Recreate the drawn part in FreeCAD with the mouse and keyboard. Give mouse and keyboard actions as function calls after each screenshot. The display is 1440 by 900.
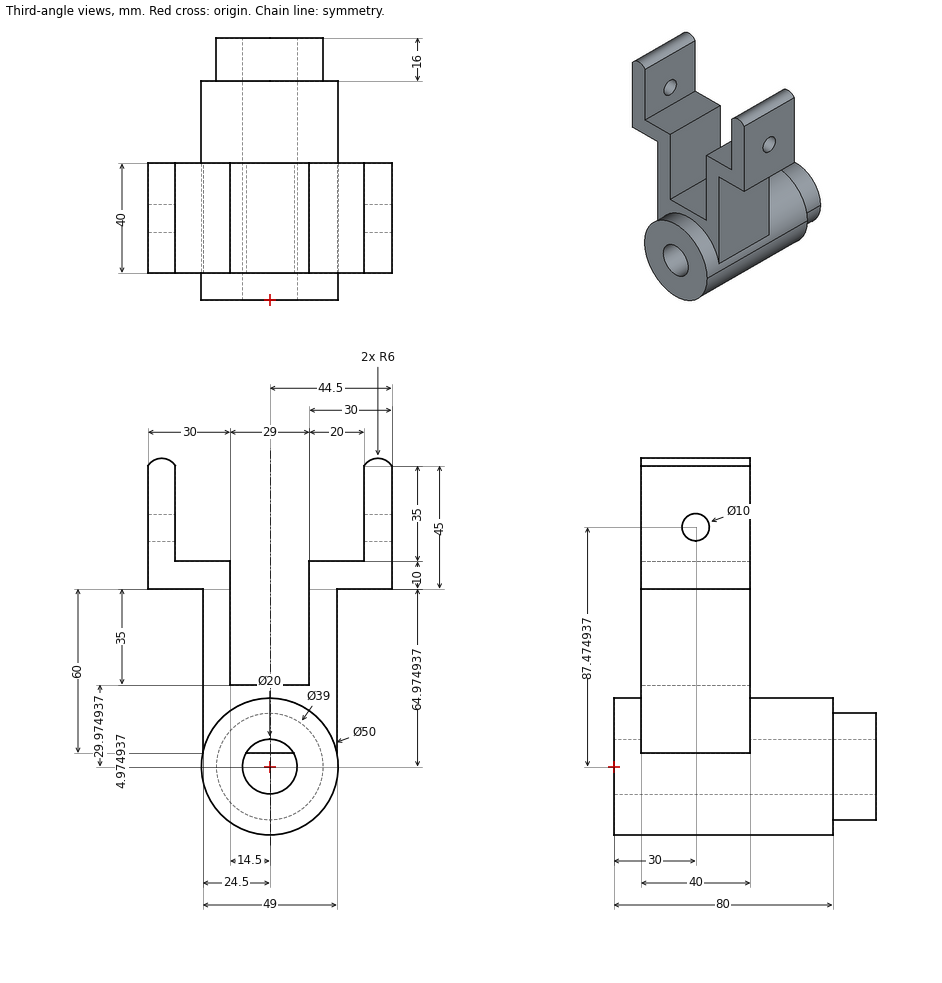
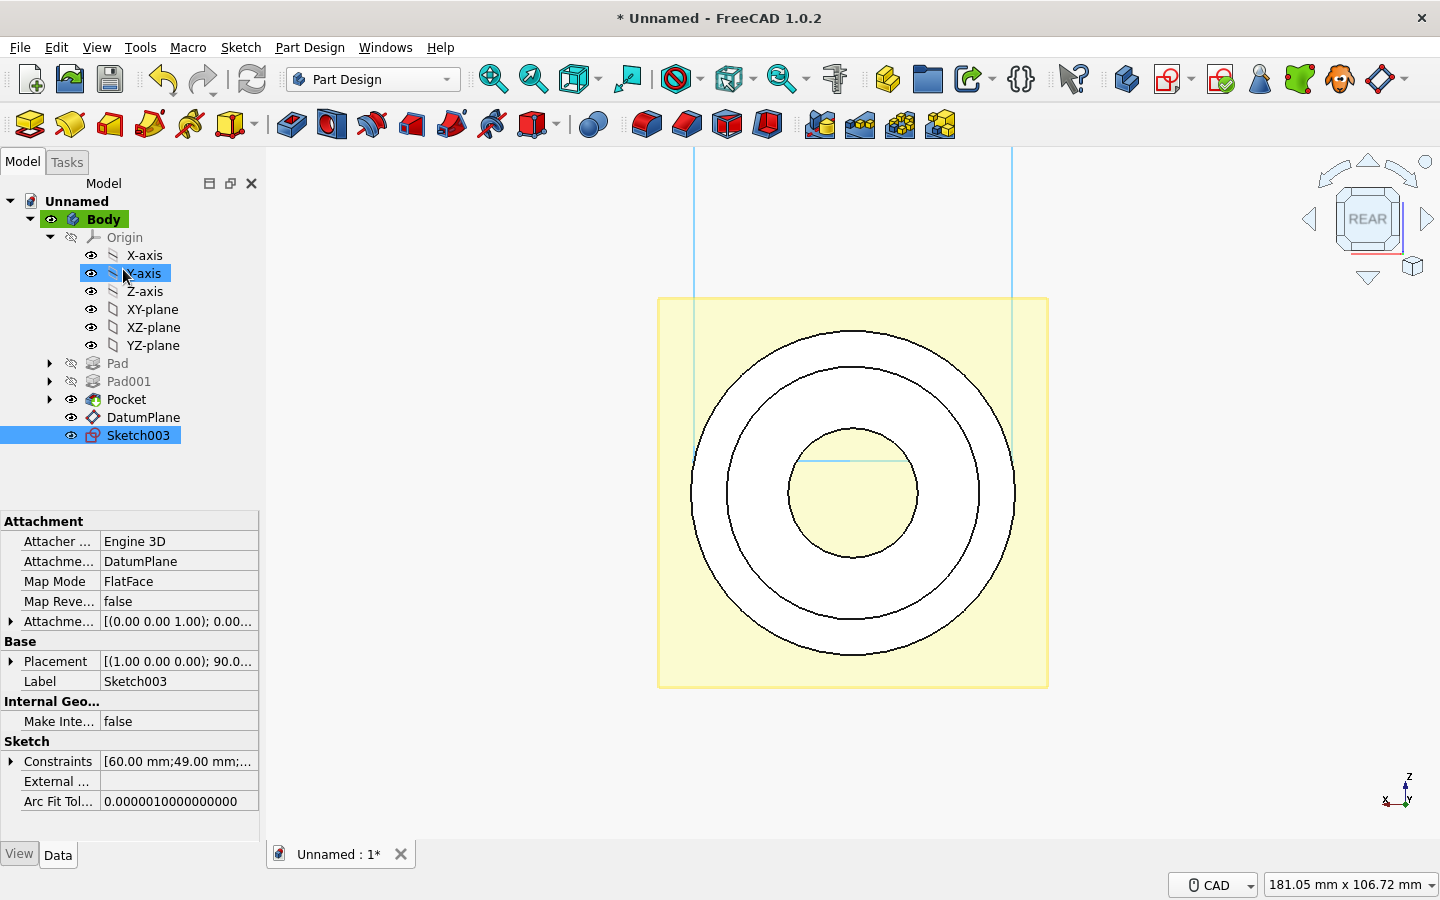
click(30, 124)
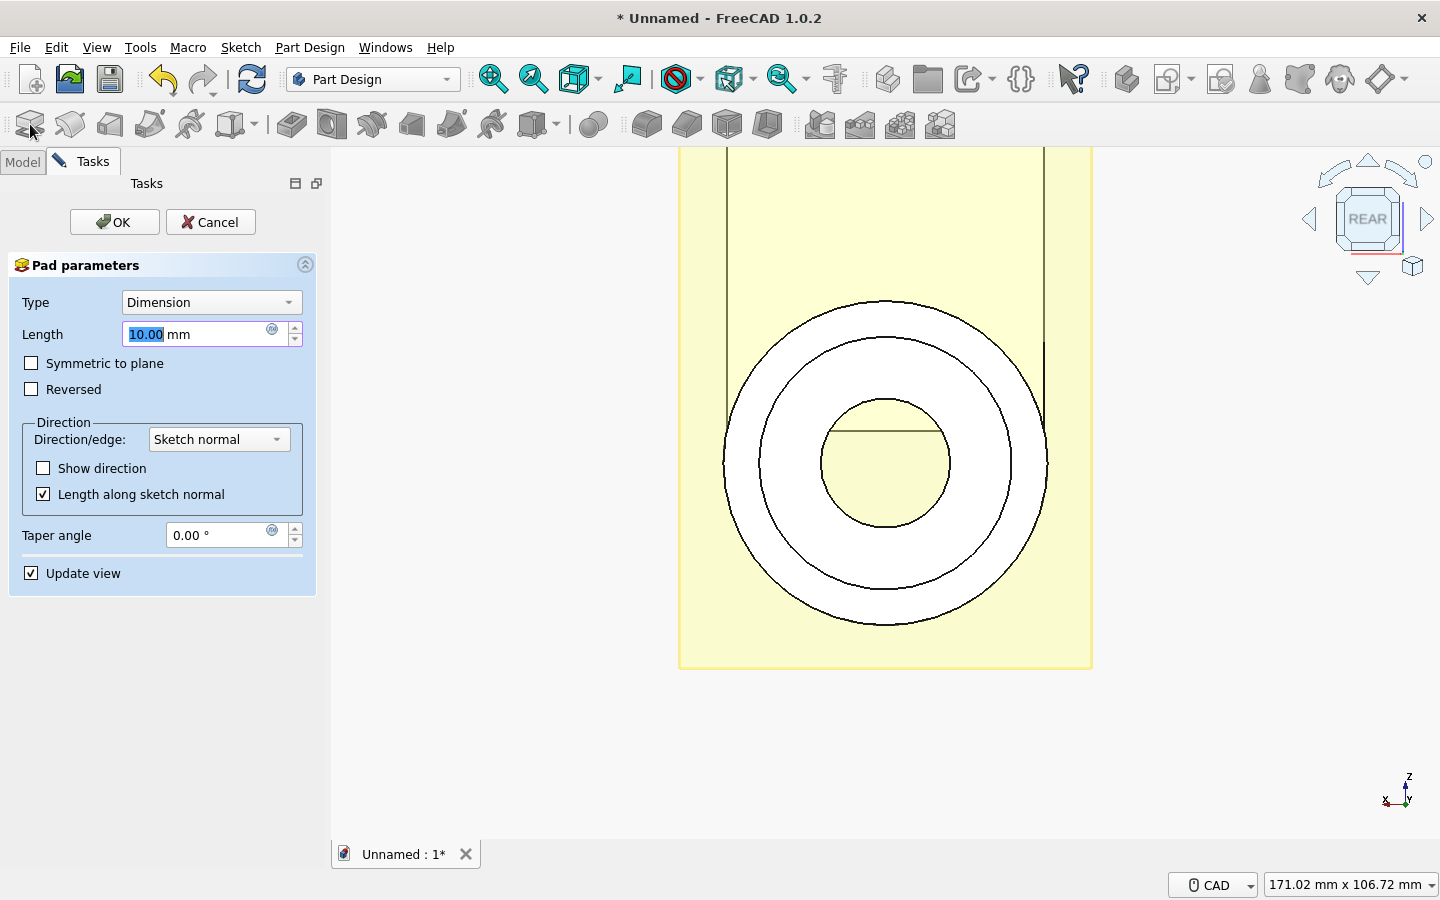
text(40)
key(Tab)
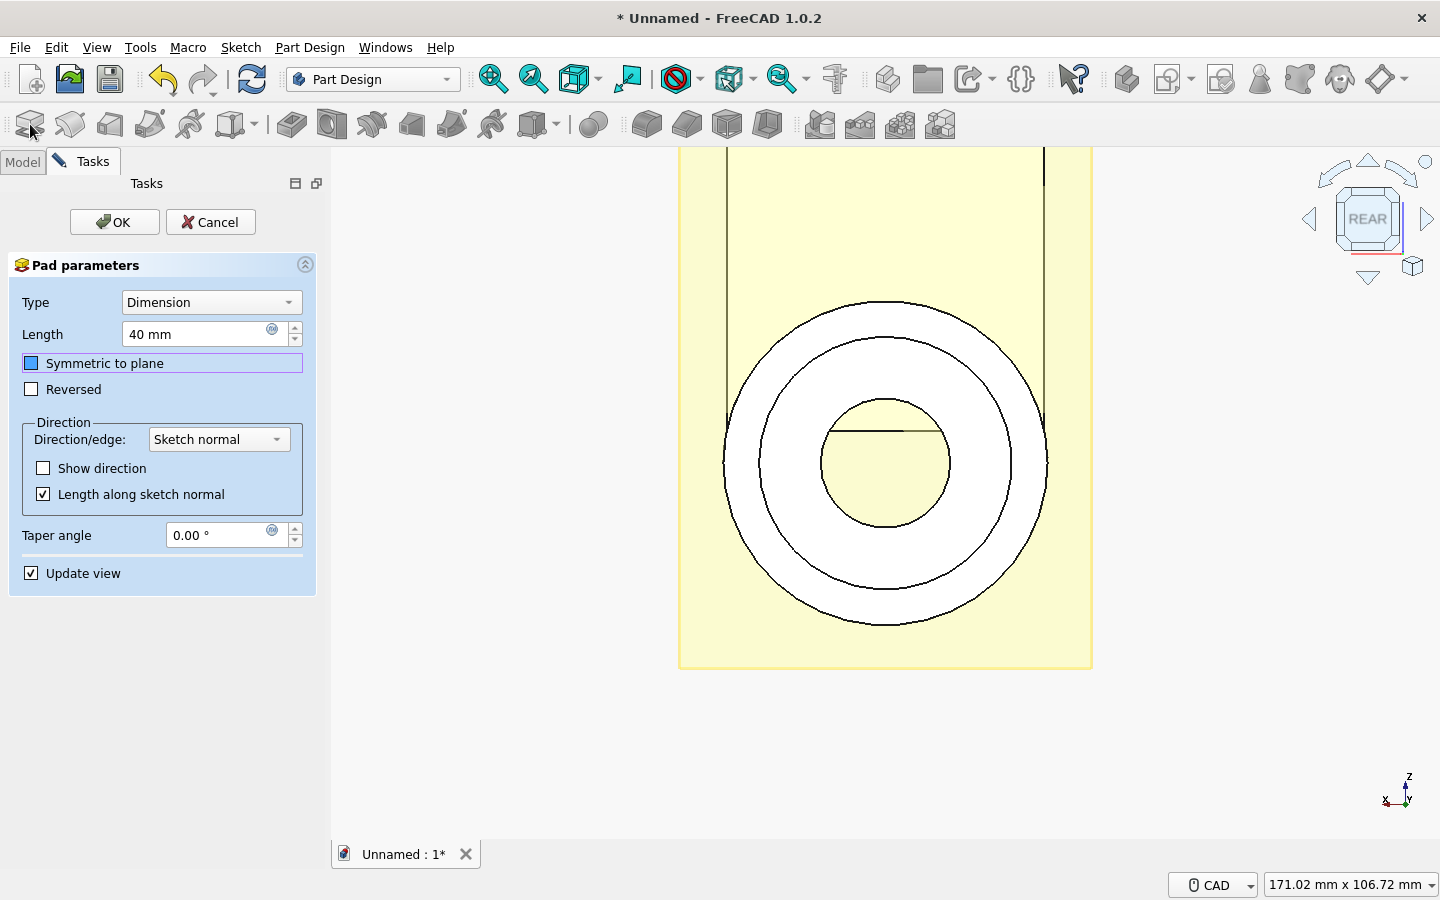
click(30, 389)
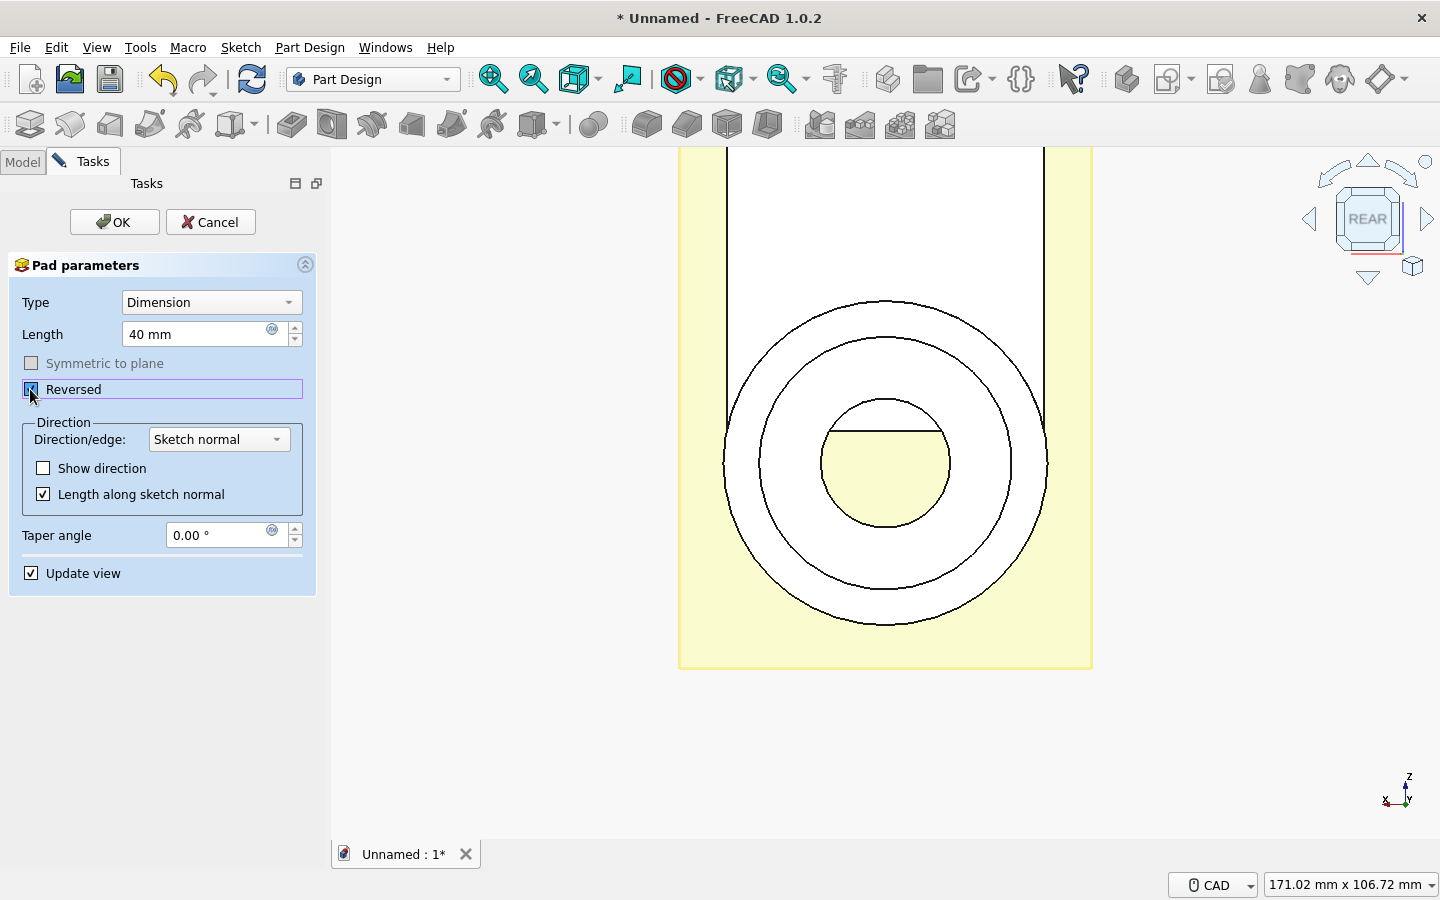
click(115, 222)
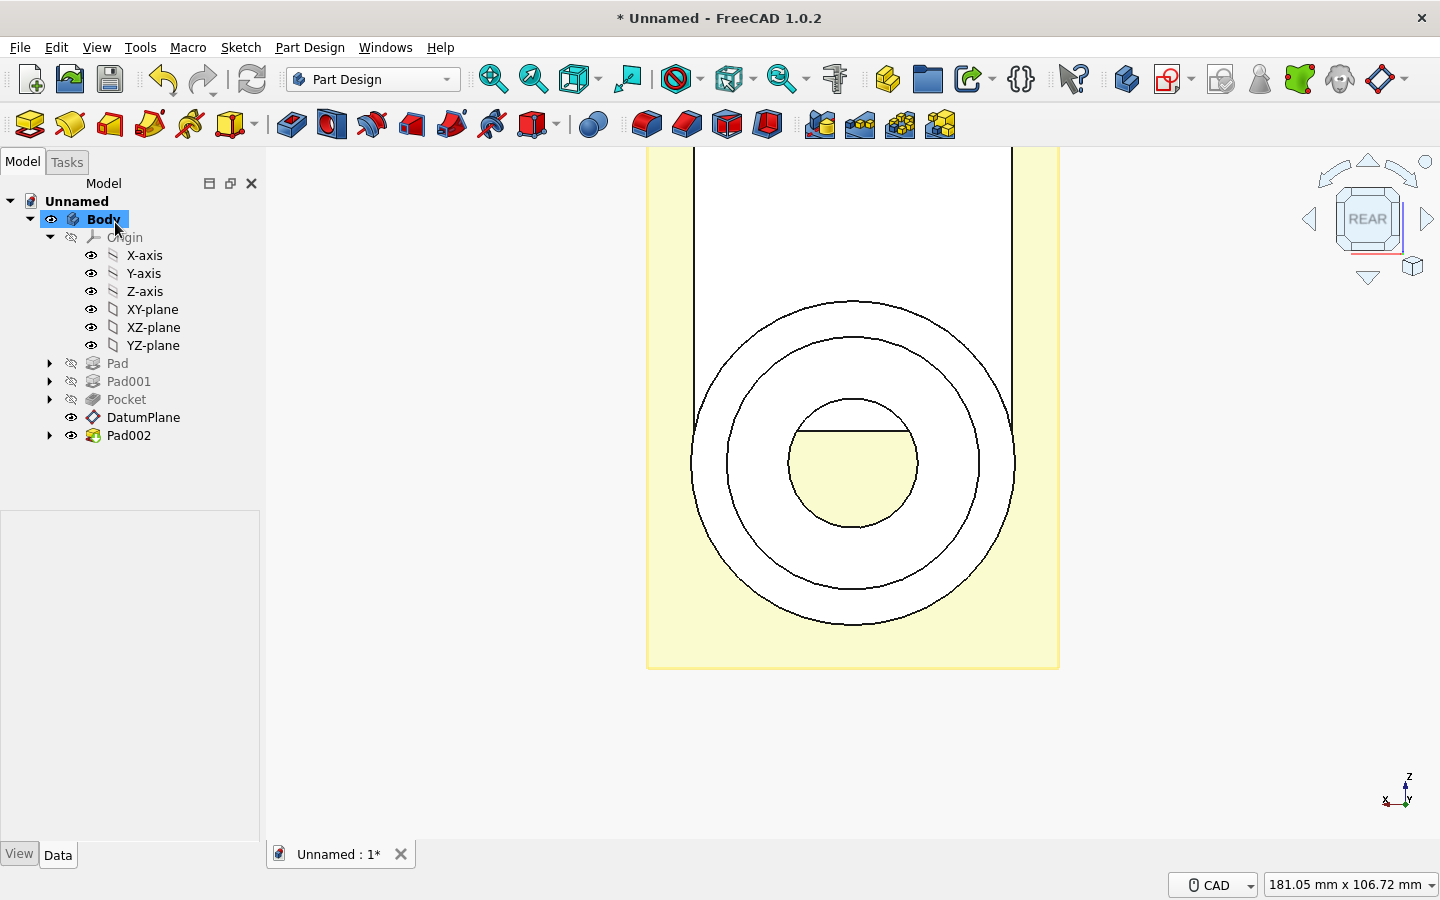
click(116, 417)
key(space)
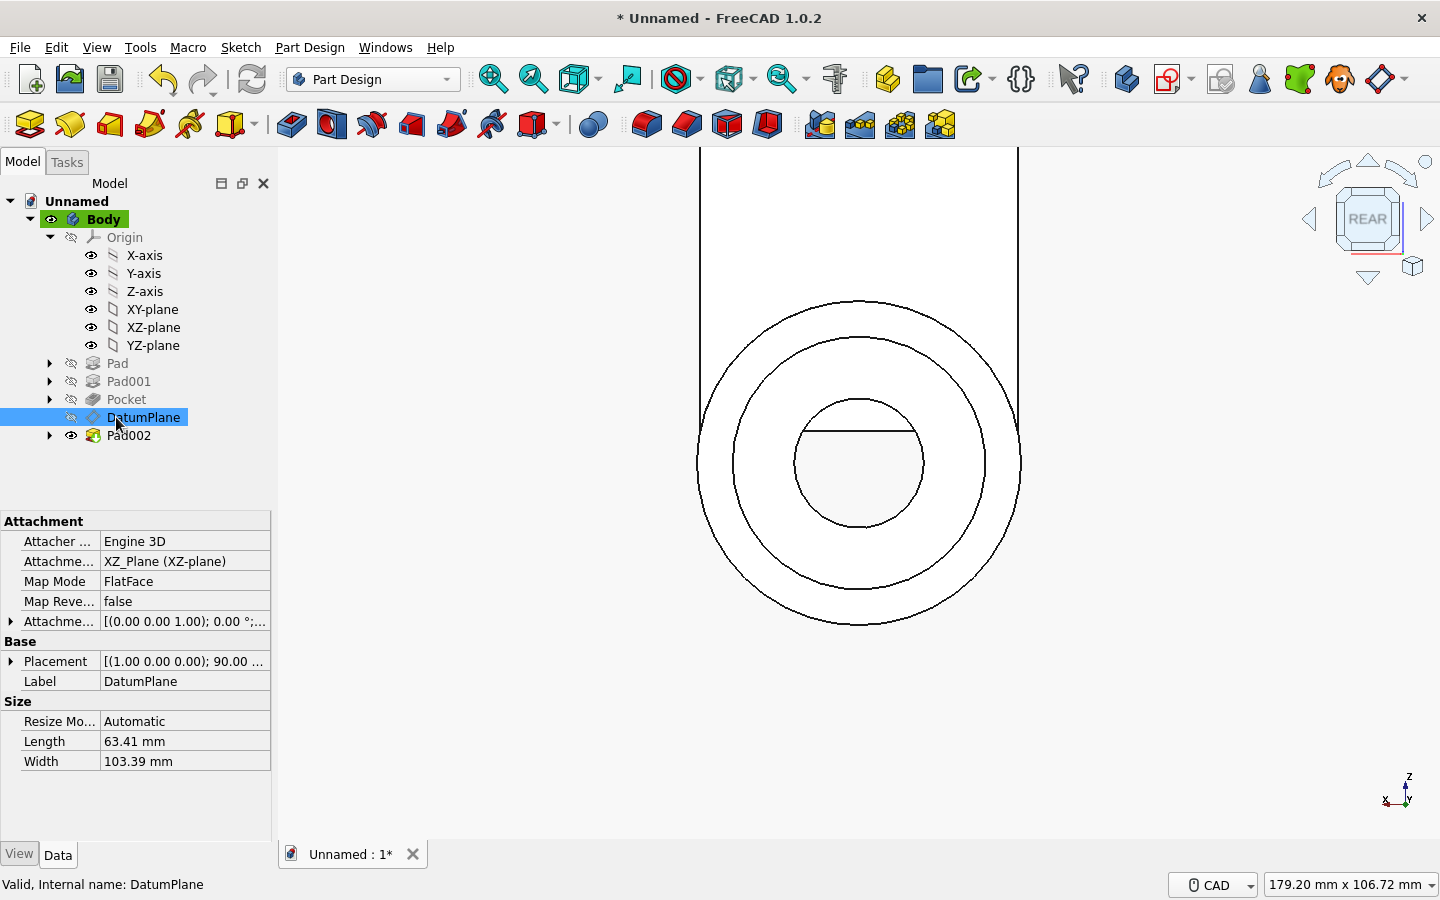
click(494, 80)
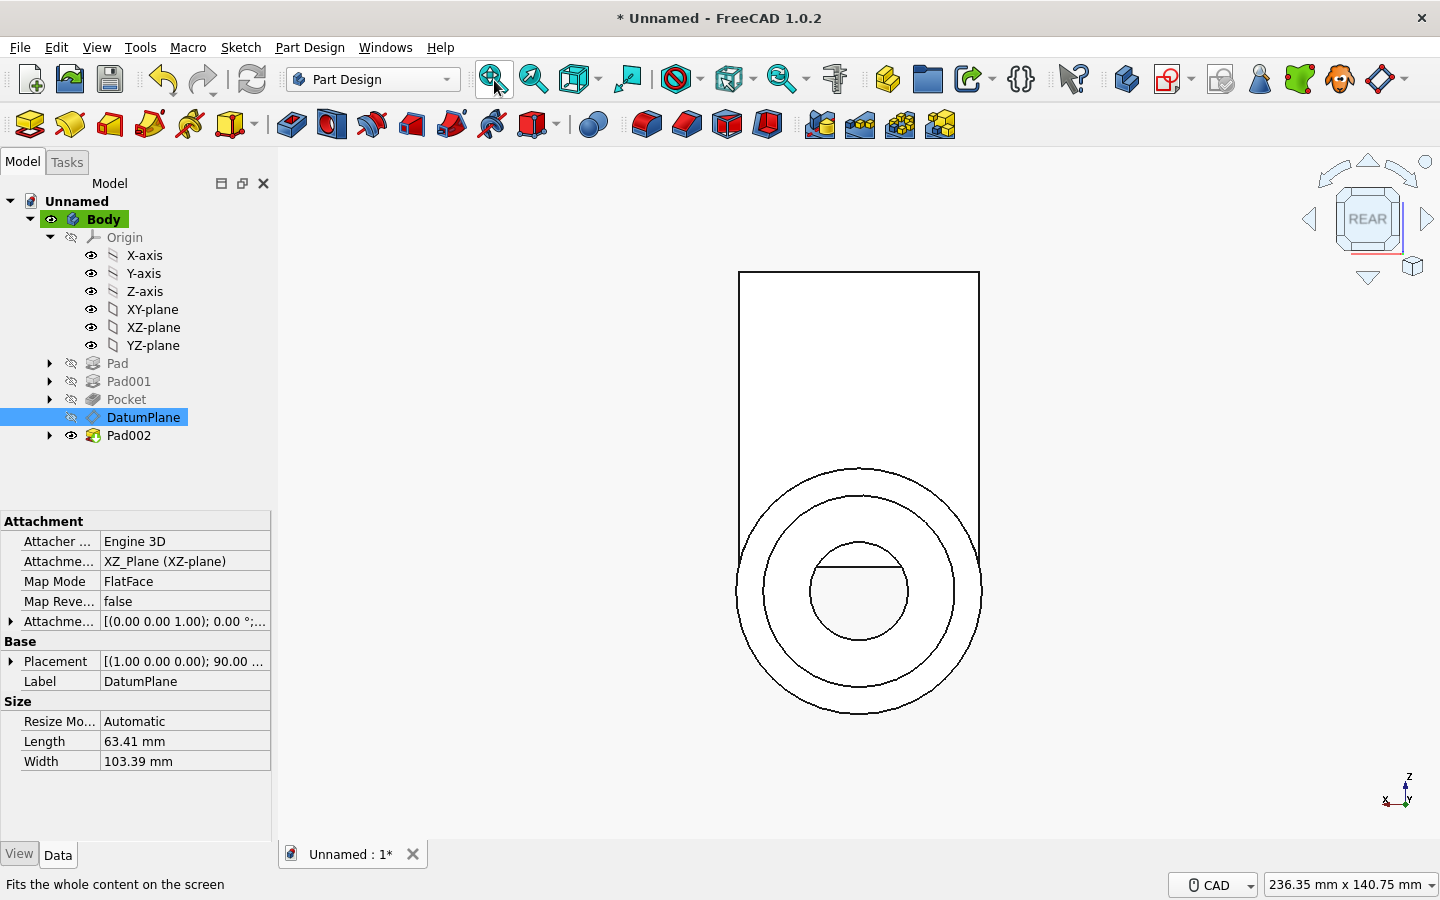
click(859, 376)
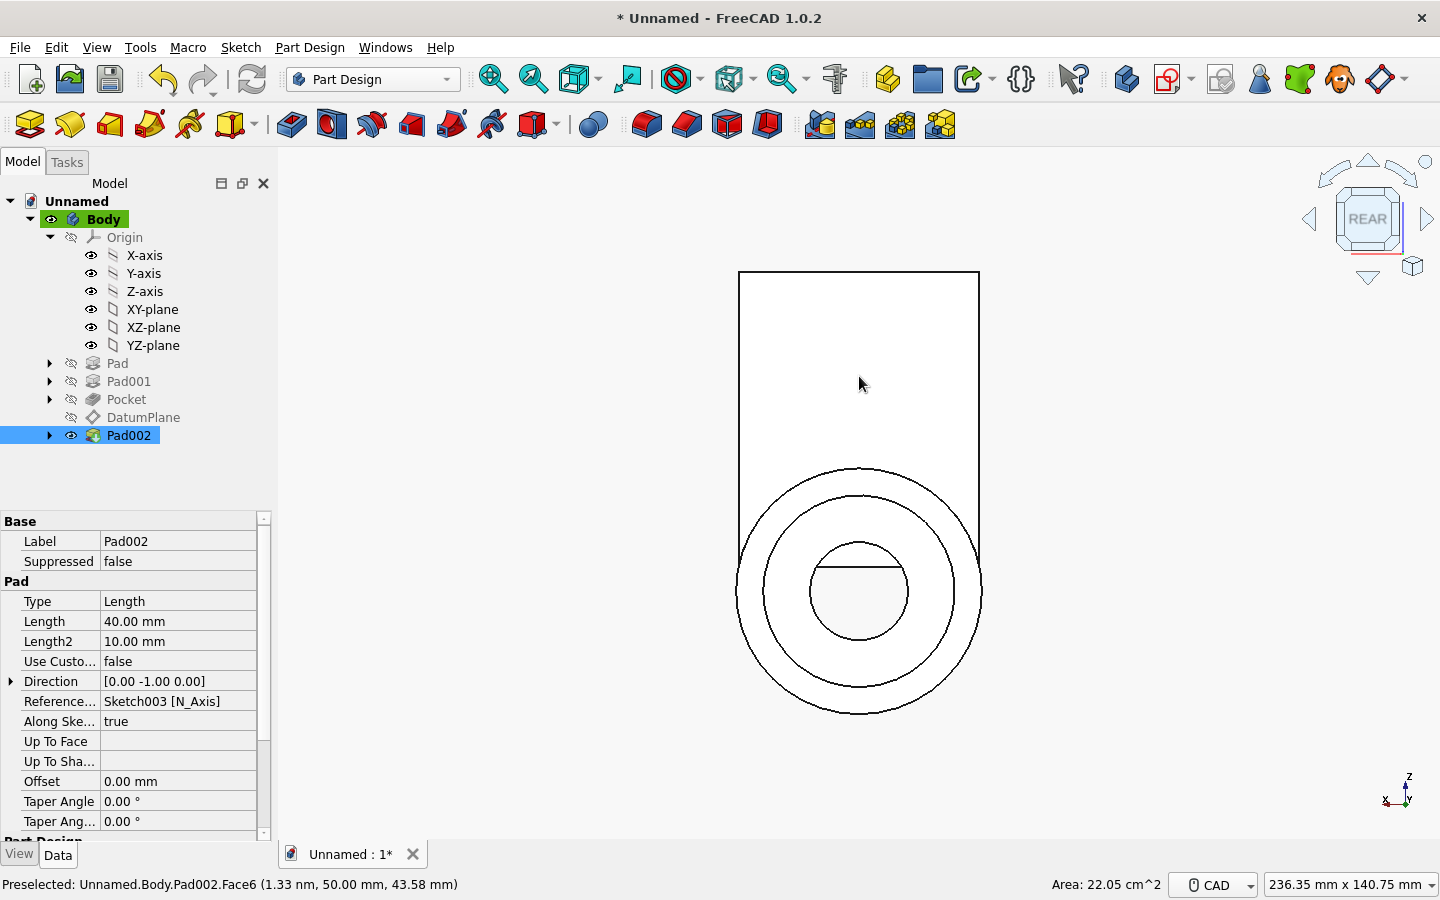
click(1168, 80)